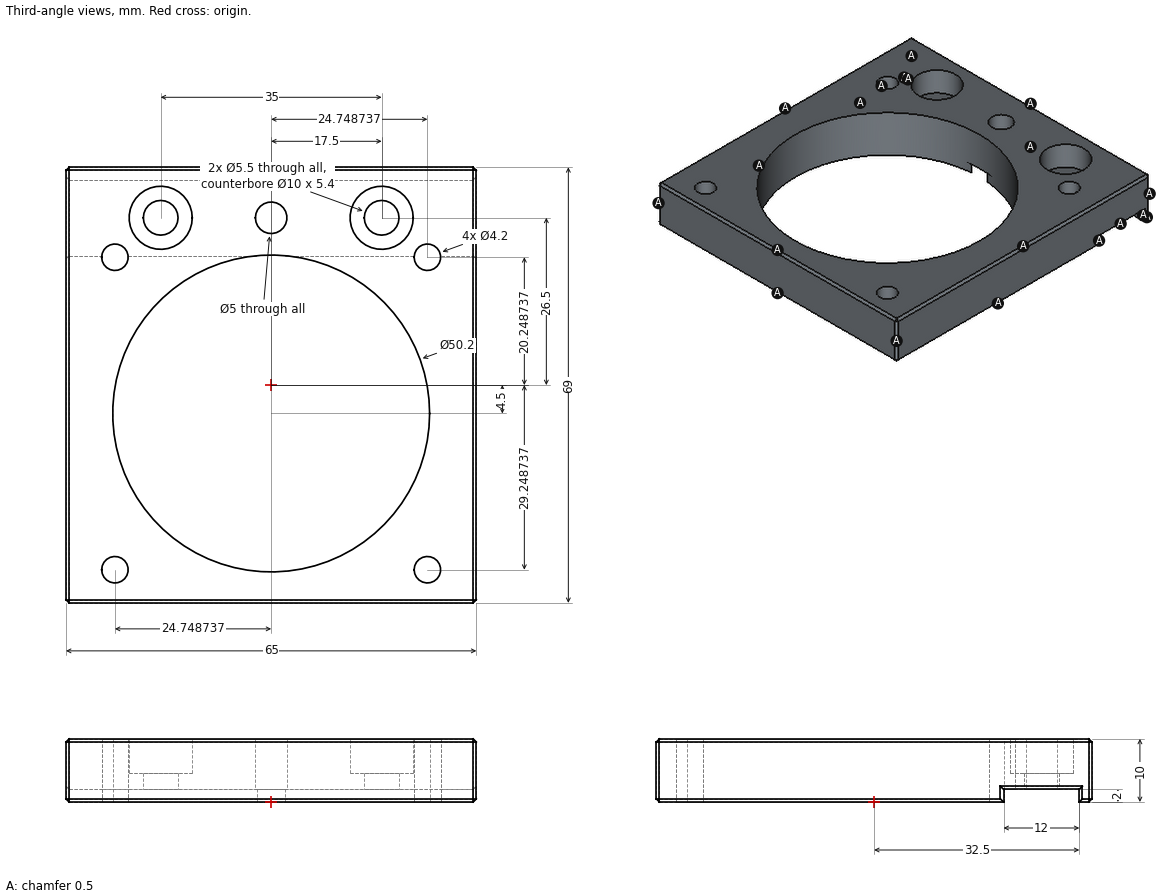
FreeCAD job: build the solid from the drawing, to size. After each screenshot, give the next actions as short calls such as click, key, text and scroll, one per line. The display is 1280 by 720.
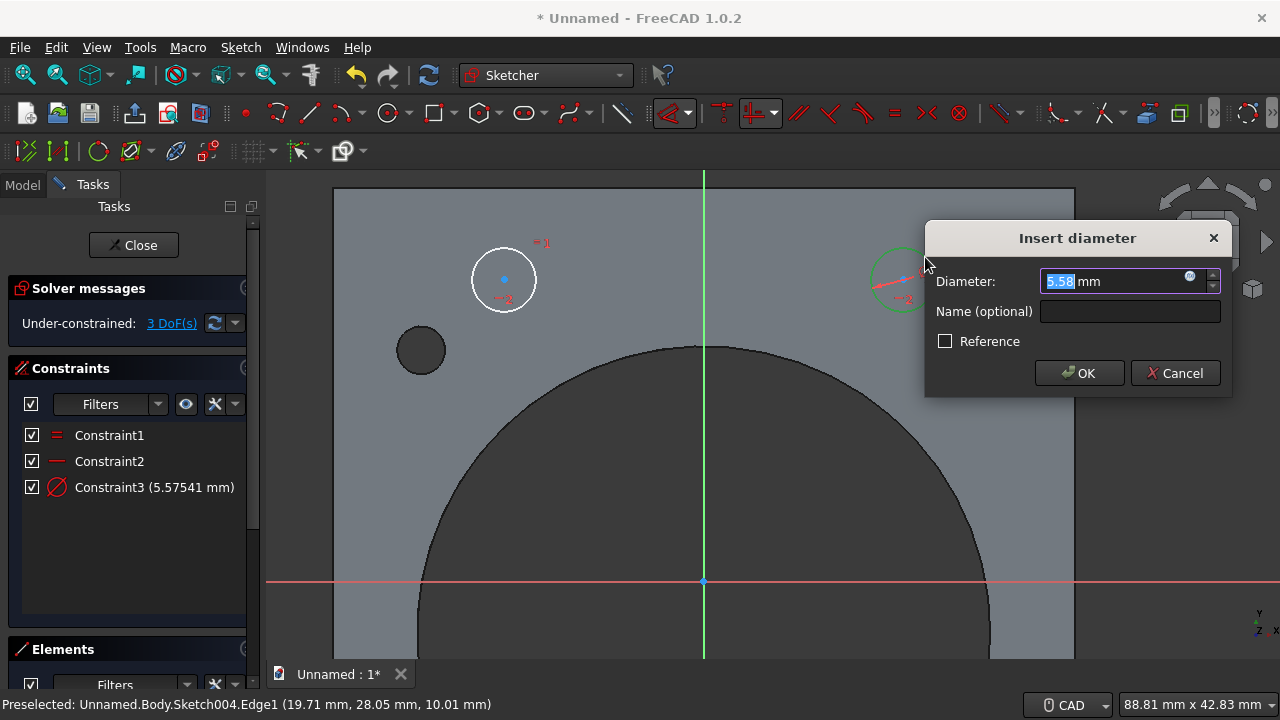
text(5.5)
key(Return)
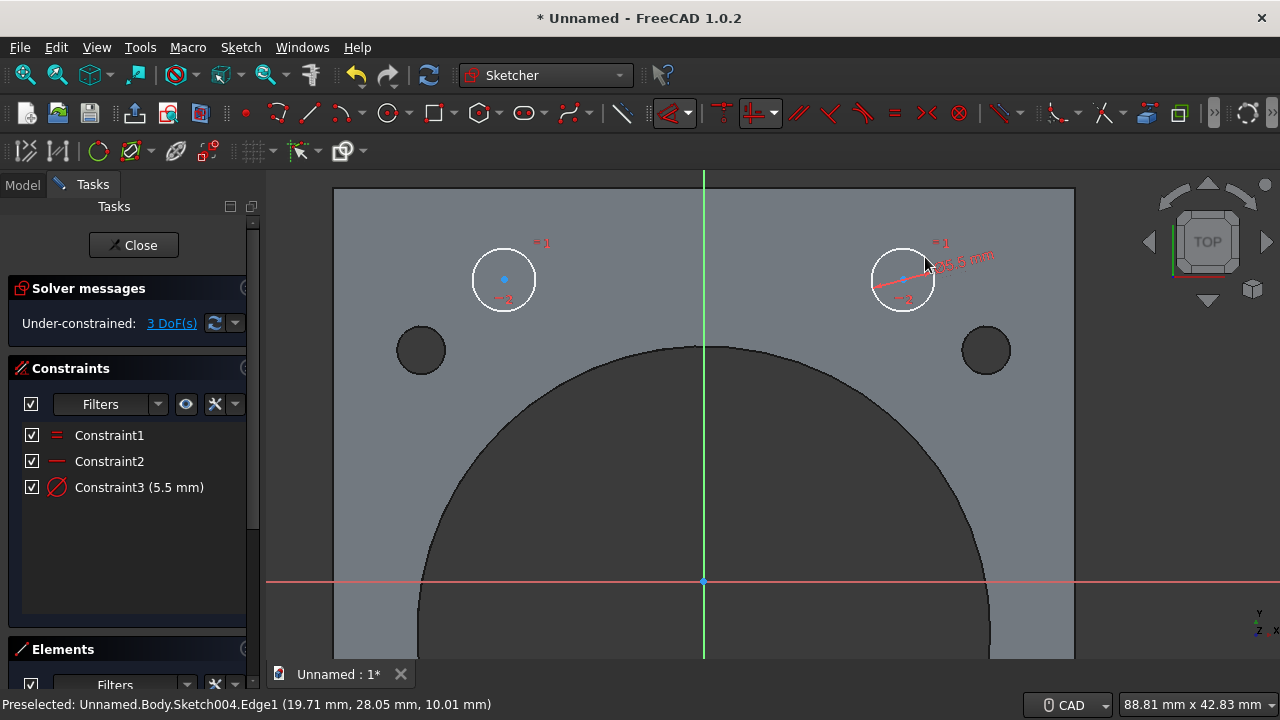
click(903, 280)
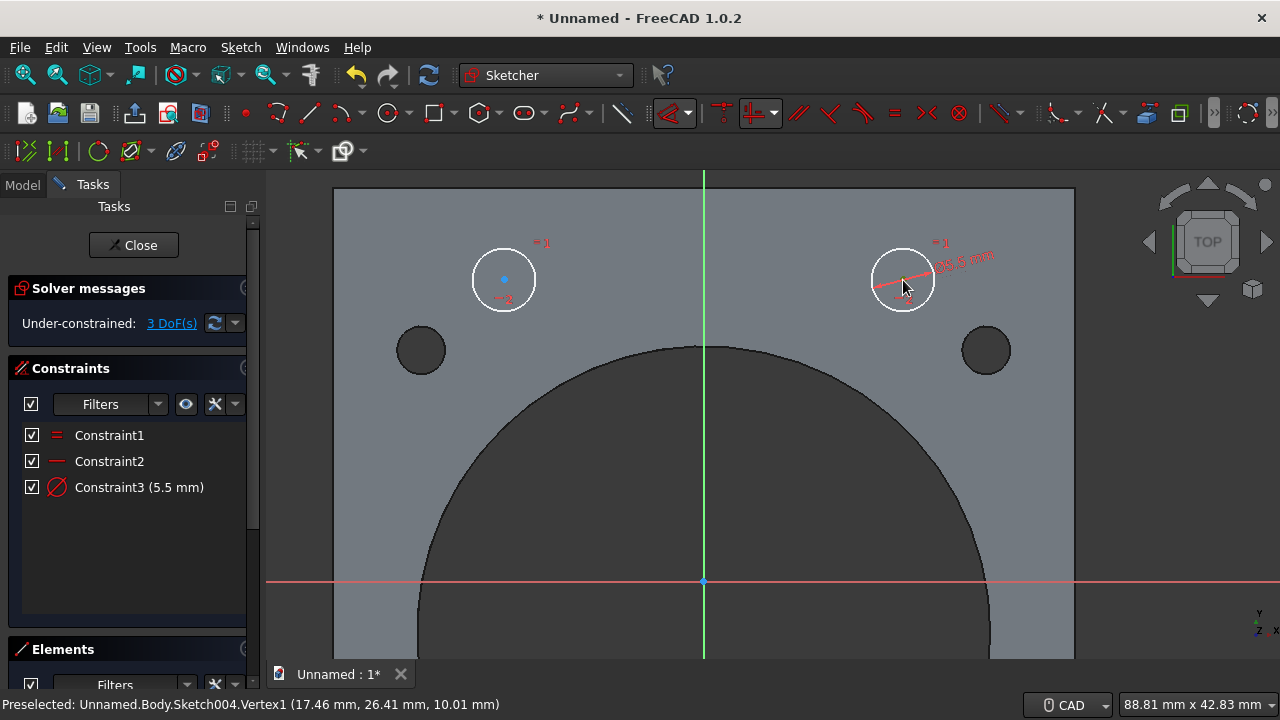
click(504, 280)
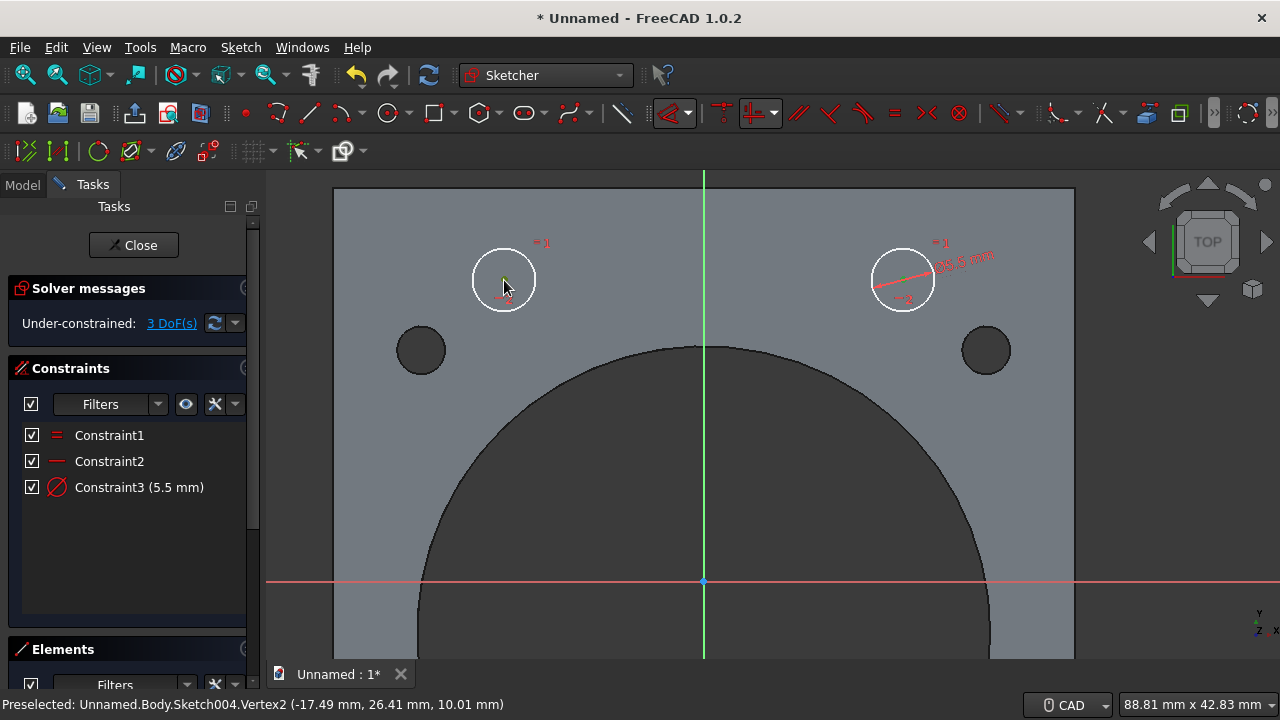
click(690, 114)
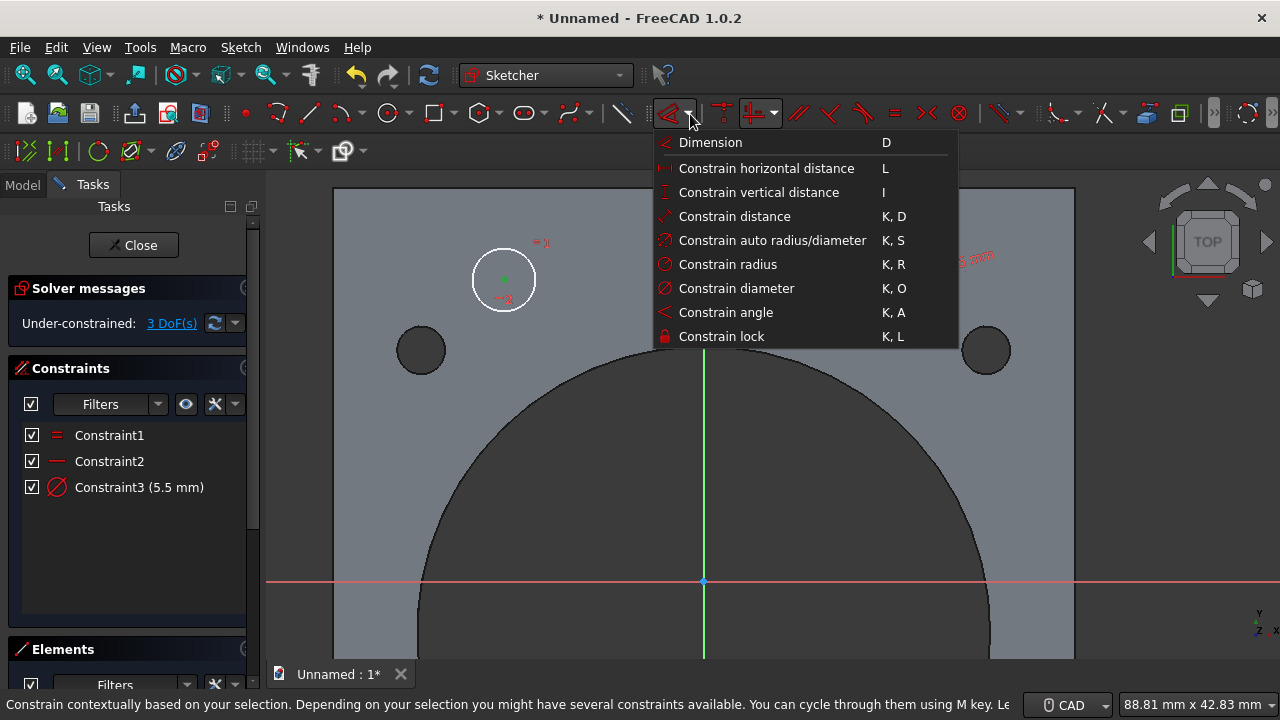
click(806, 168)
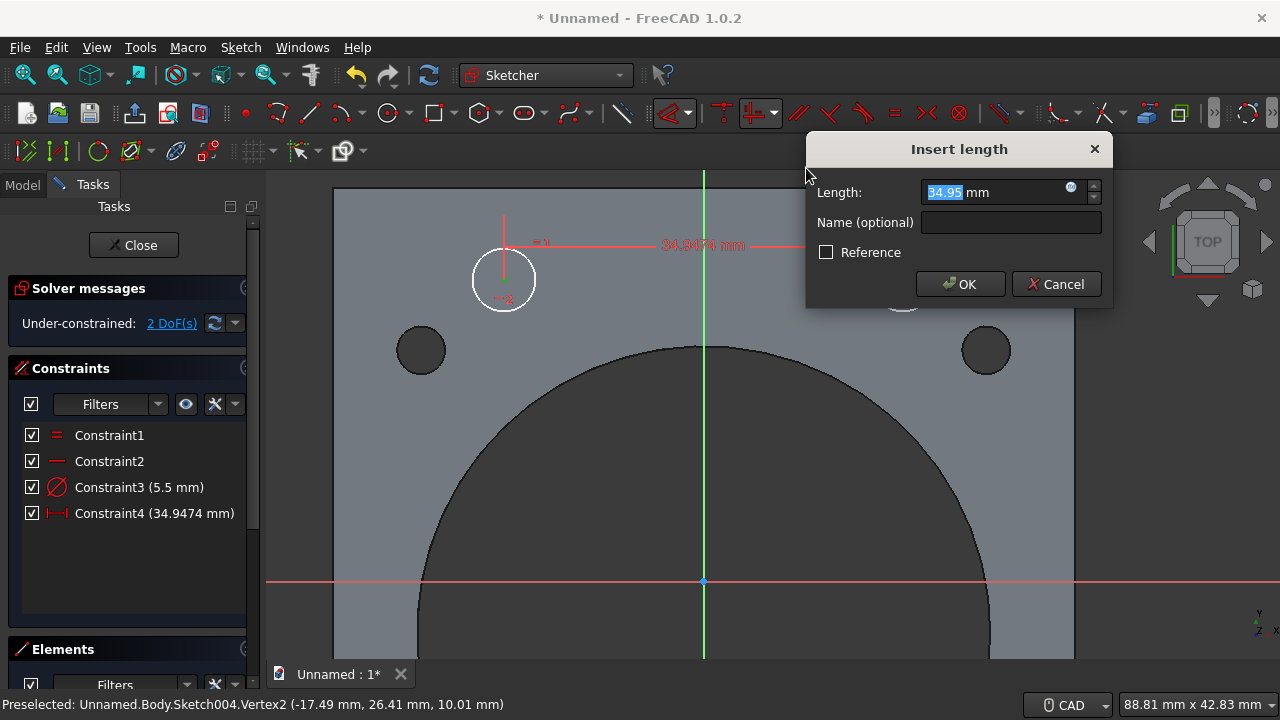
text(35)
key(Return)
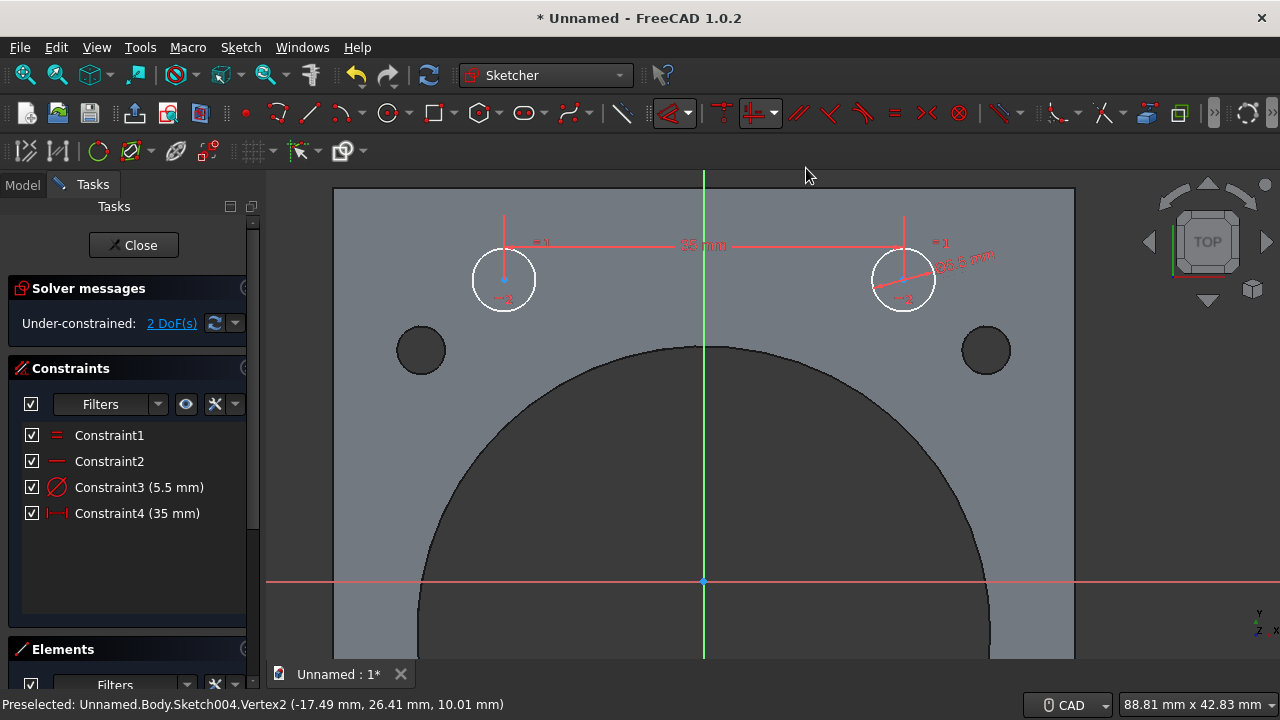
click(904, 280)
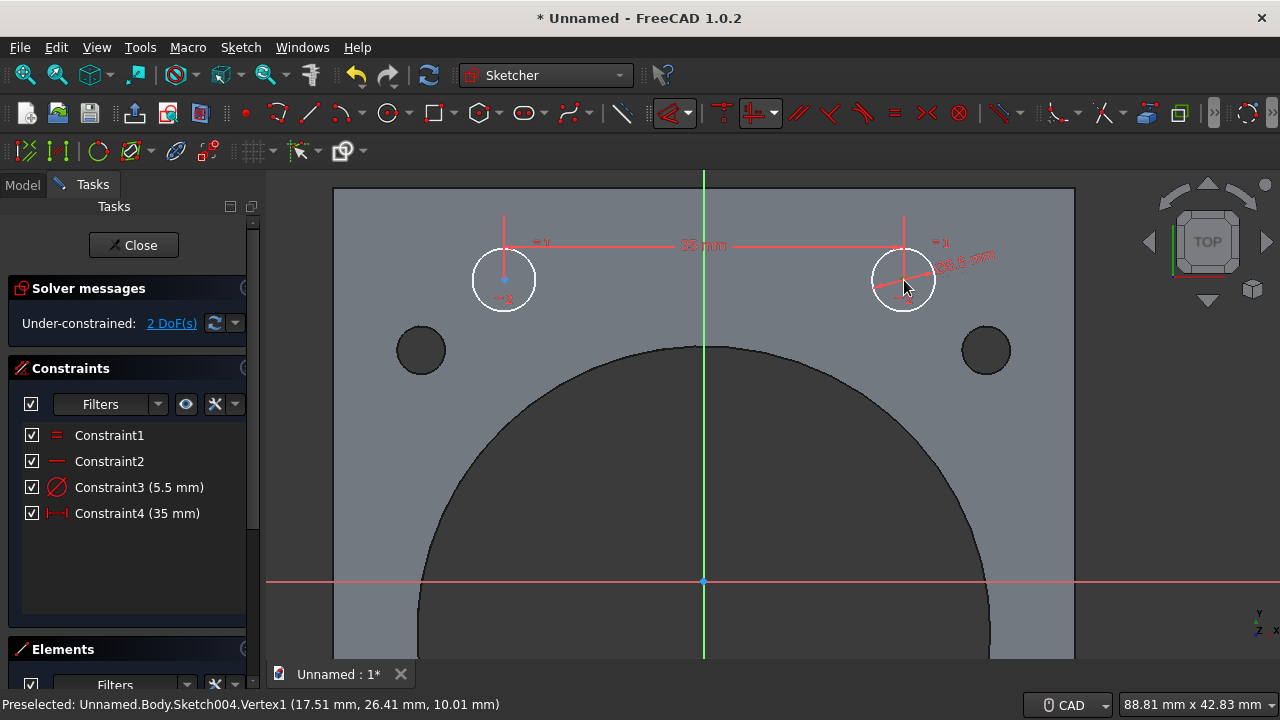
click(690, 114)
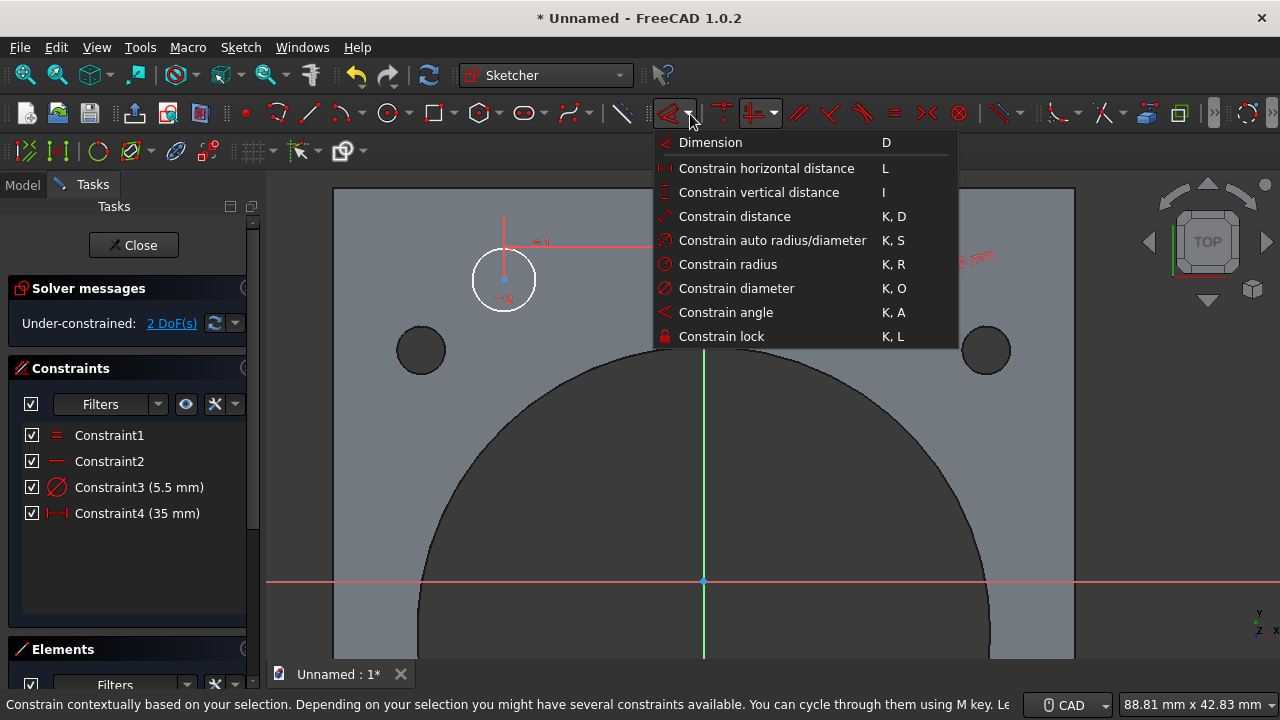
click(806, 168)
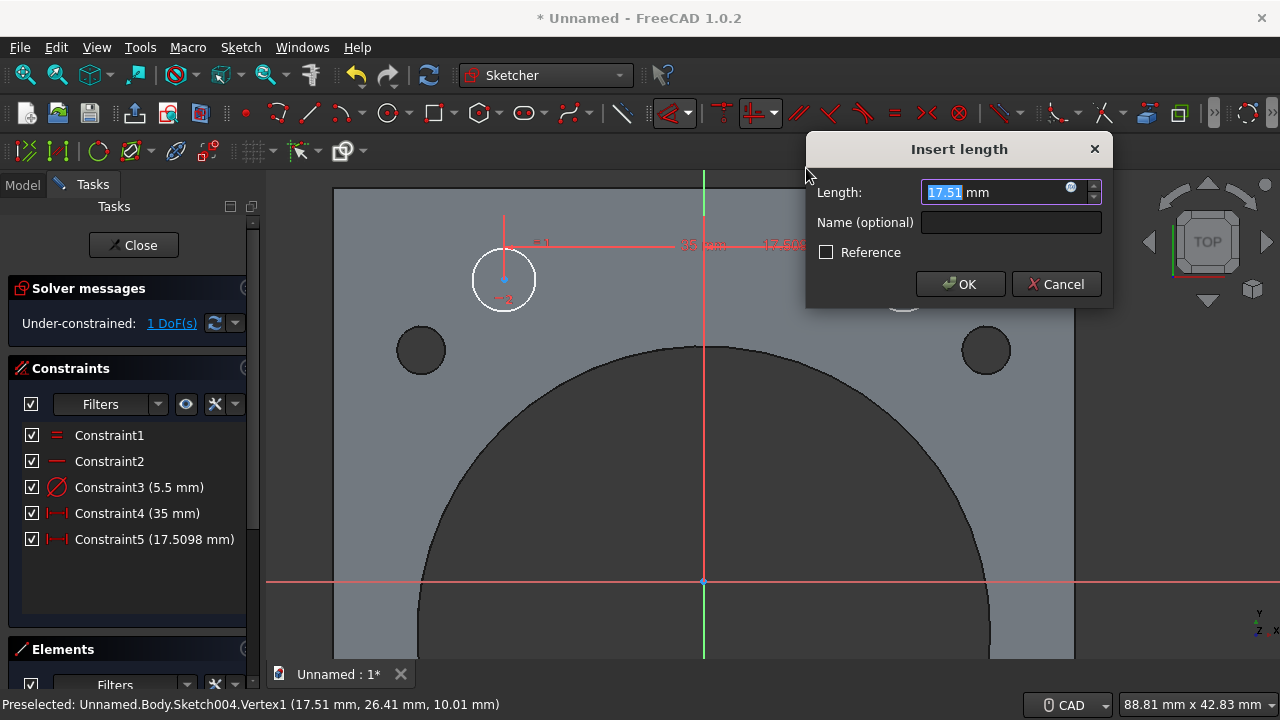
text(17.5)
key(Return)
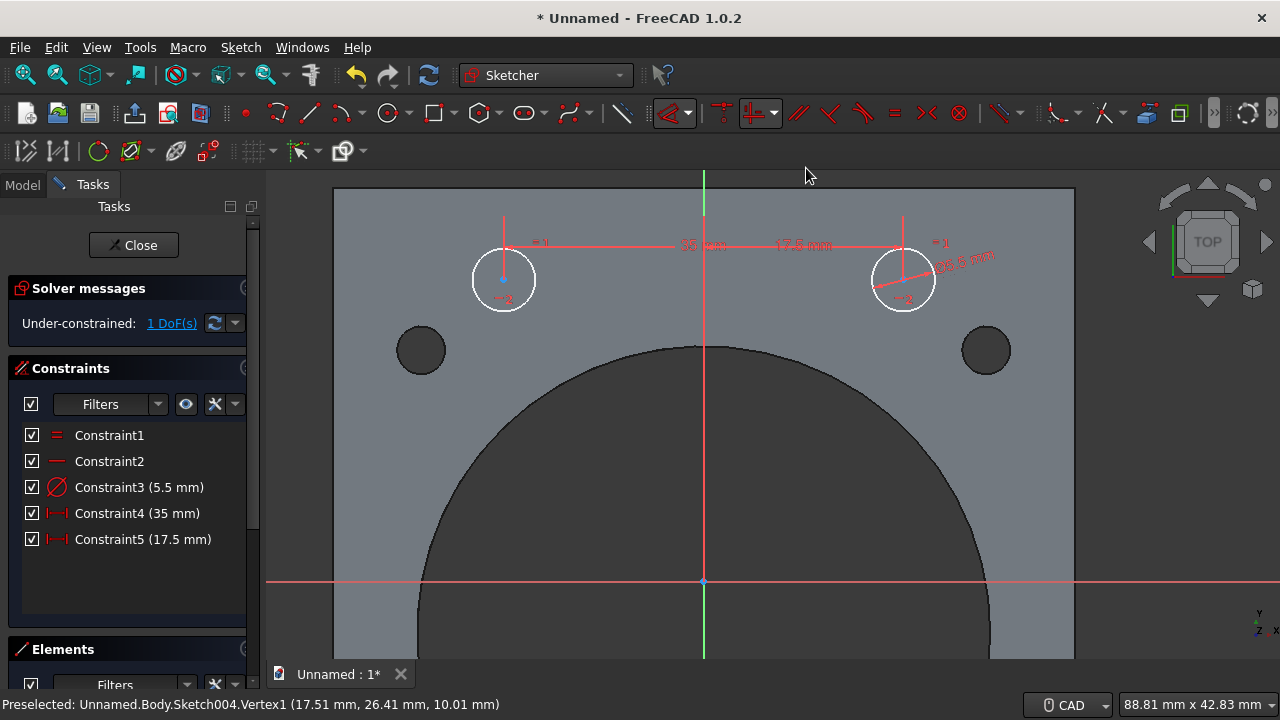
click(903, 280)